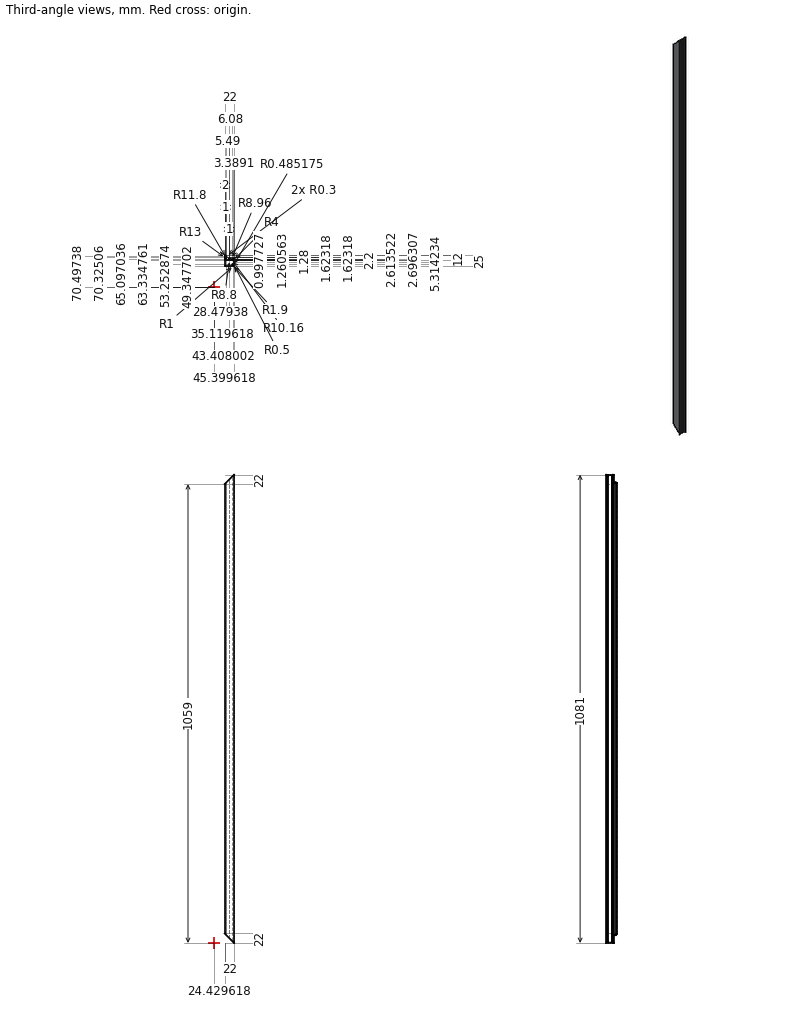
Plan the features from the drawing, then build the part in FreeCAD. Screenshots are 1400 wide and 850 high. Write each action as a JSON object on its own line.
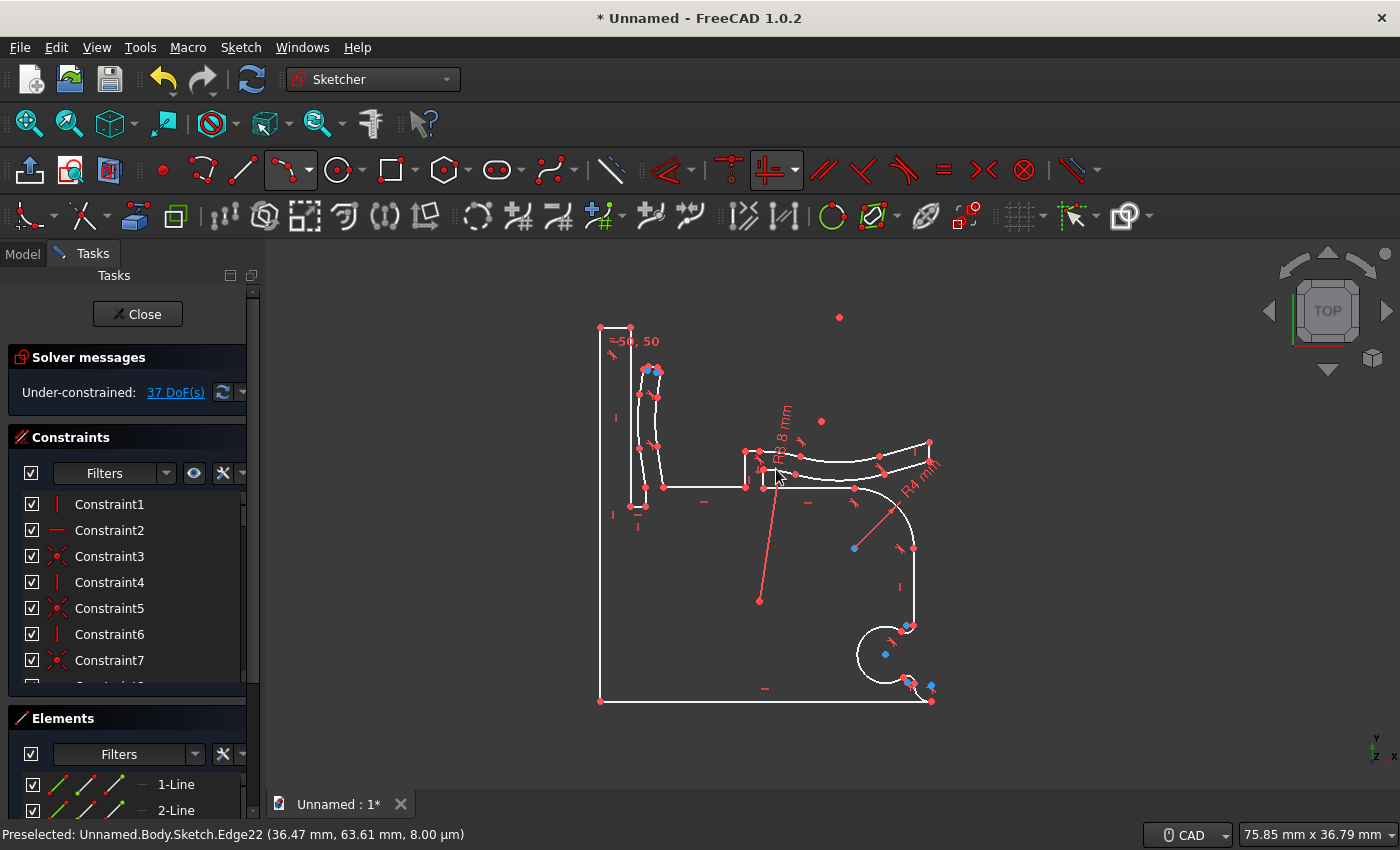
{"action": "scroll", "coordinate": [813, 478], "scroll_direction": "up", "scroll_amount": 2}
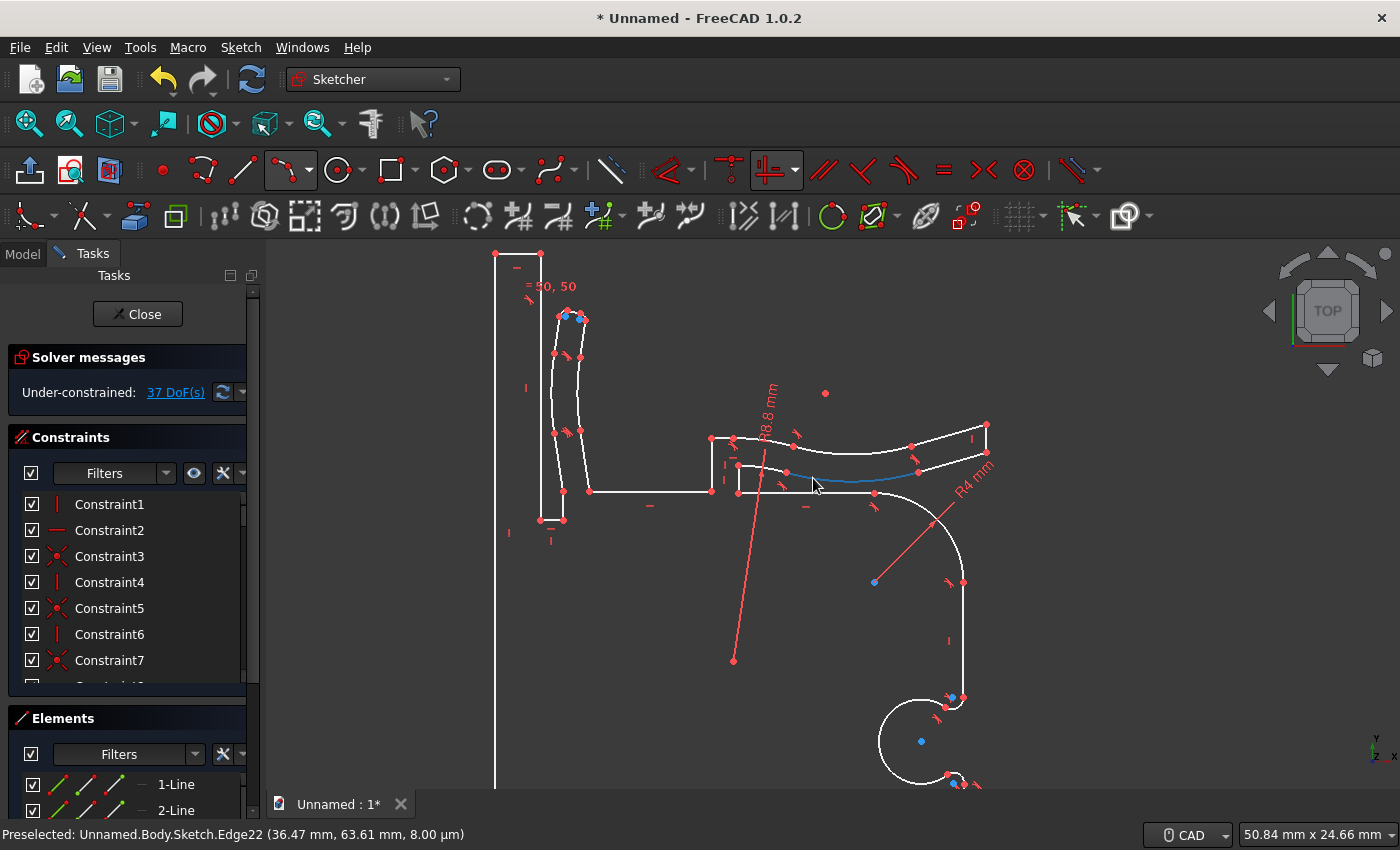
{"action": "left_click", "coordinate": [812, 478]}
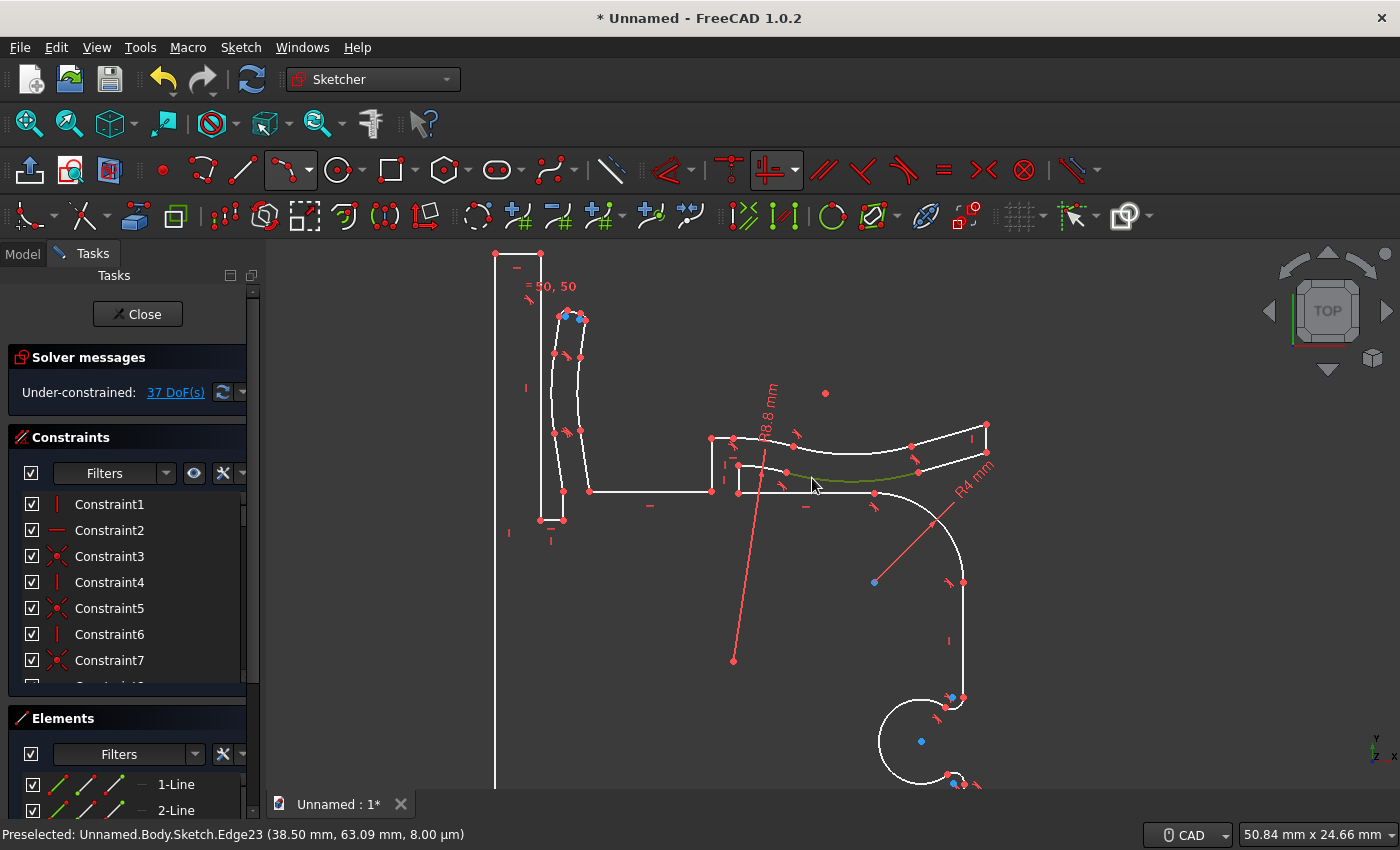
{"action": "left_click", "coordinate": [694, 170]}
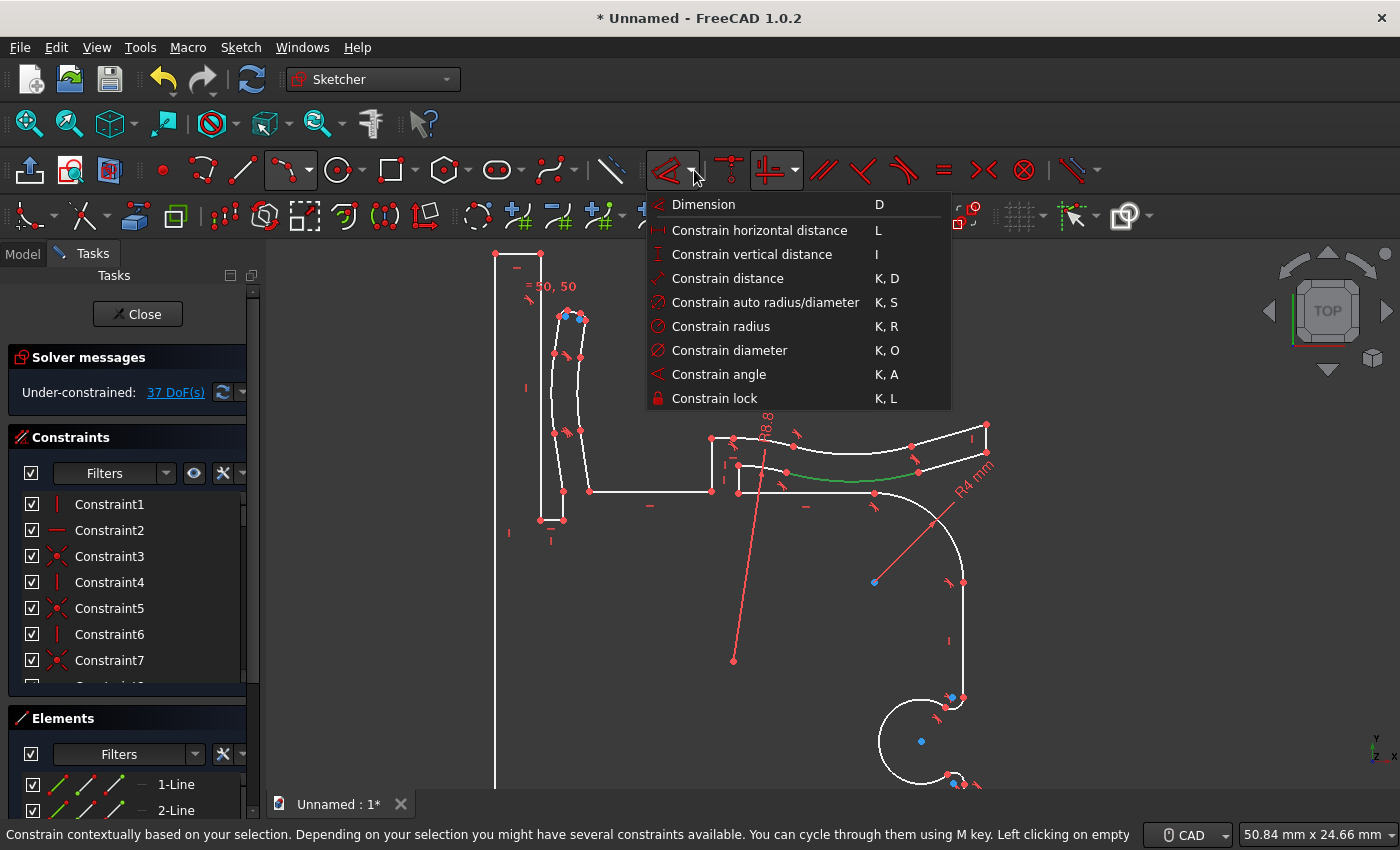
{"action": "left_click", "coordinate": [799, 326]}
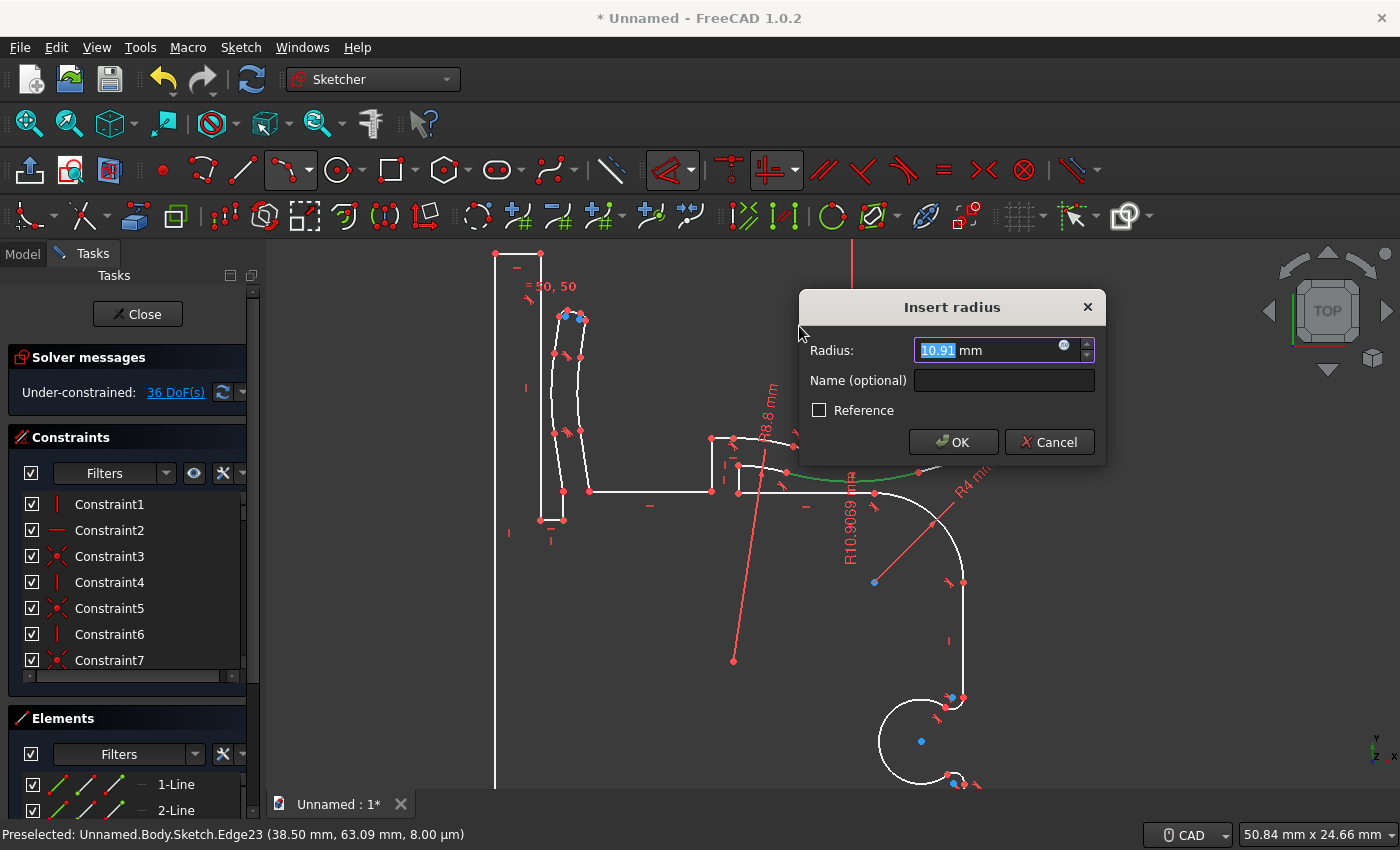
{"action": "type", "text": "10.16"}
{"action": "key", "text": "Return"}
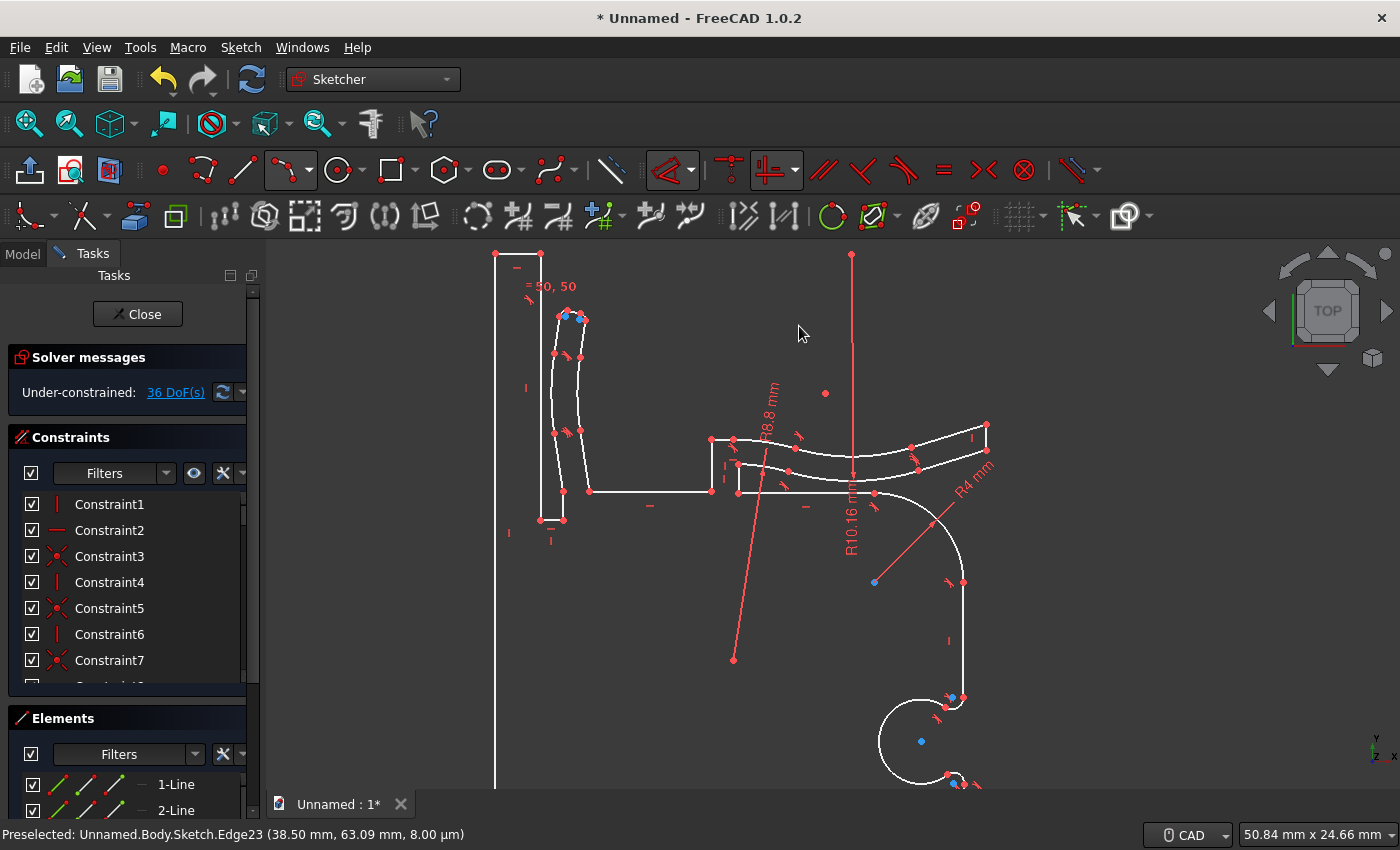
{"action": "left_click", "coordinate": [830, 455]}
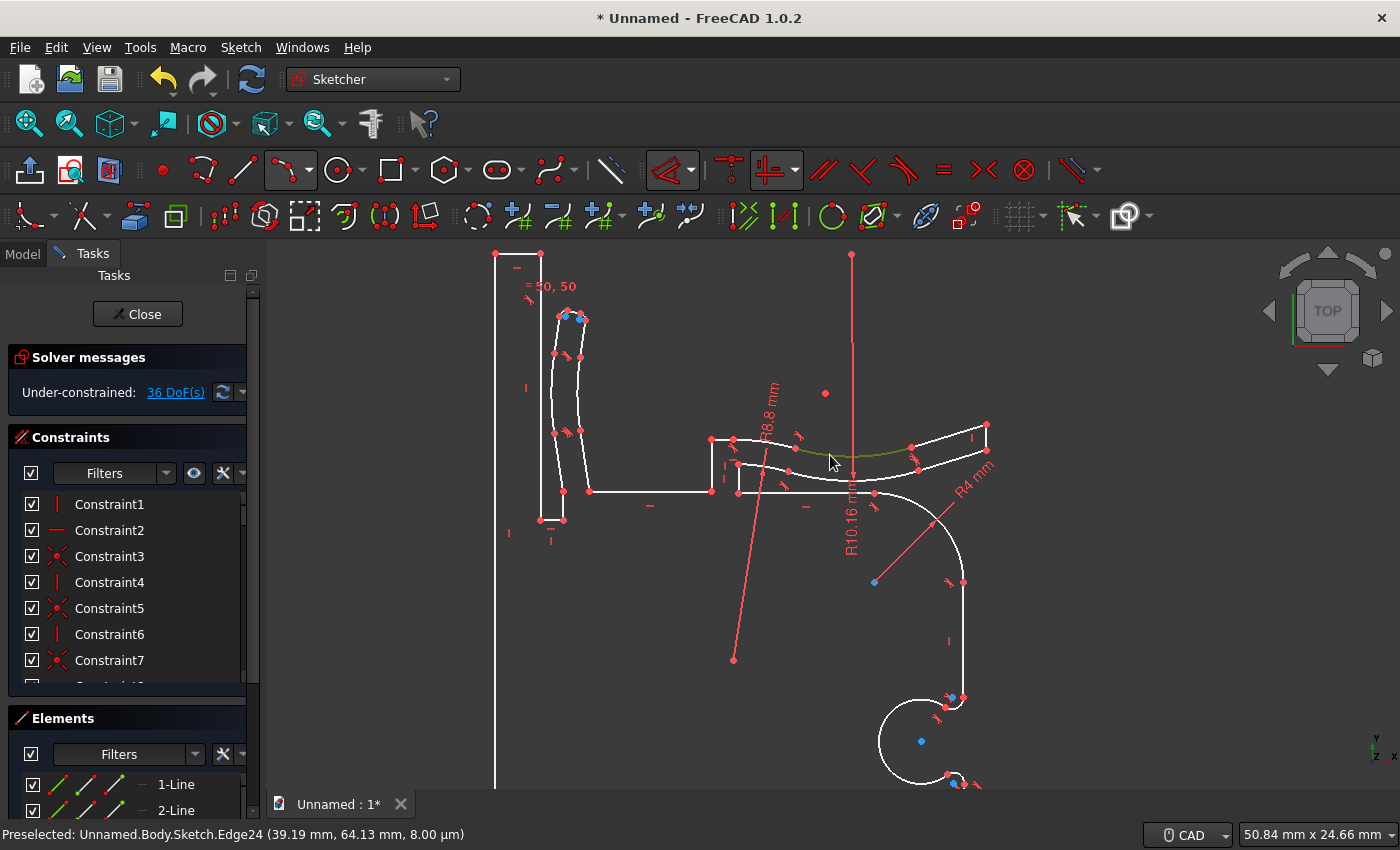
{"action": "left_click", "coordinate": [694, 170]}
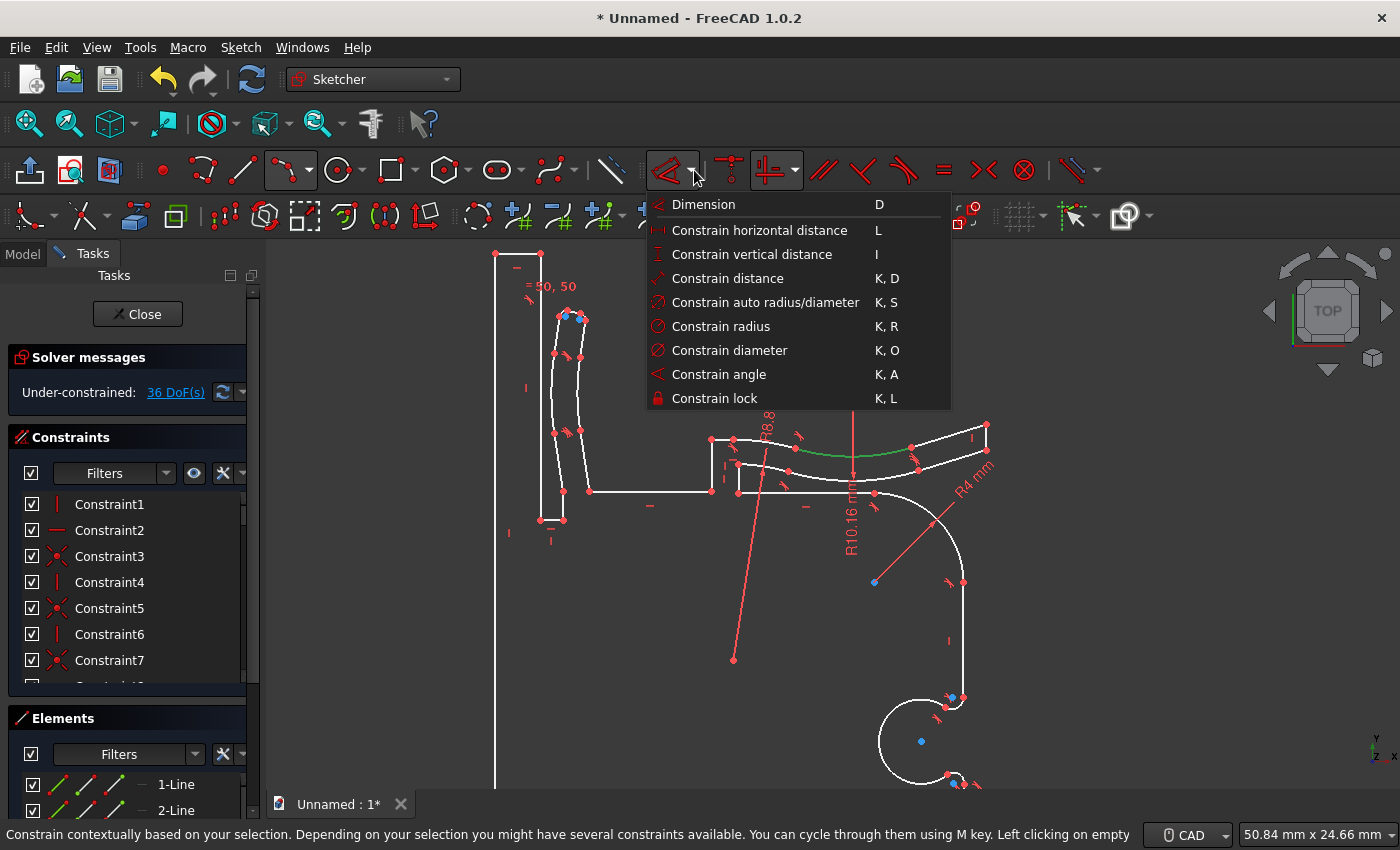
{"action": "left_click", "coordinate": [799, 326]}